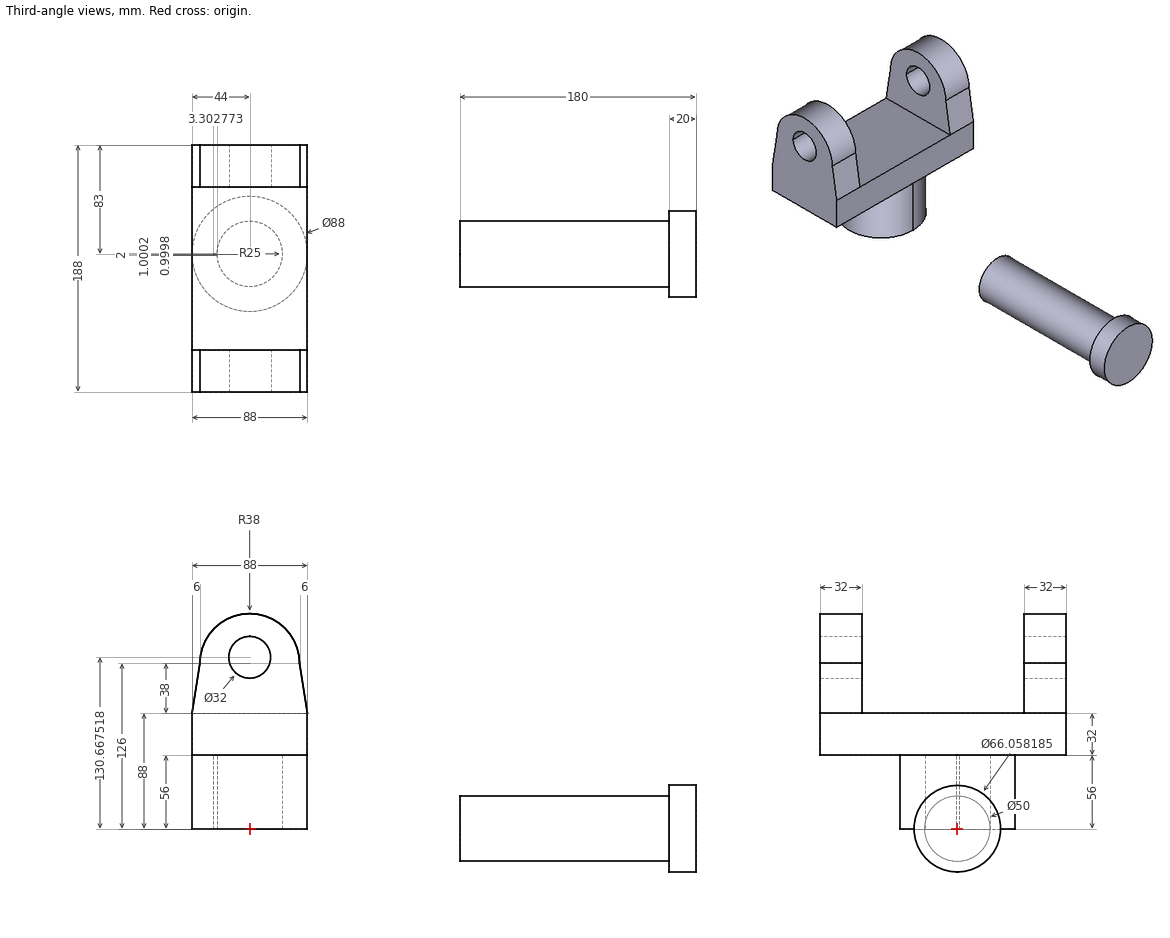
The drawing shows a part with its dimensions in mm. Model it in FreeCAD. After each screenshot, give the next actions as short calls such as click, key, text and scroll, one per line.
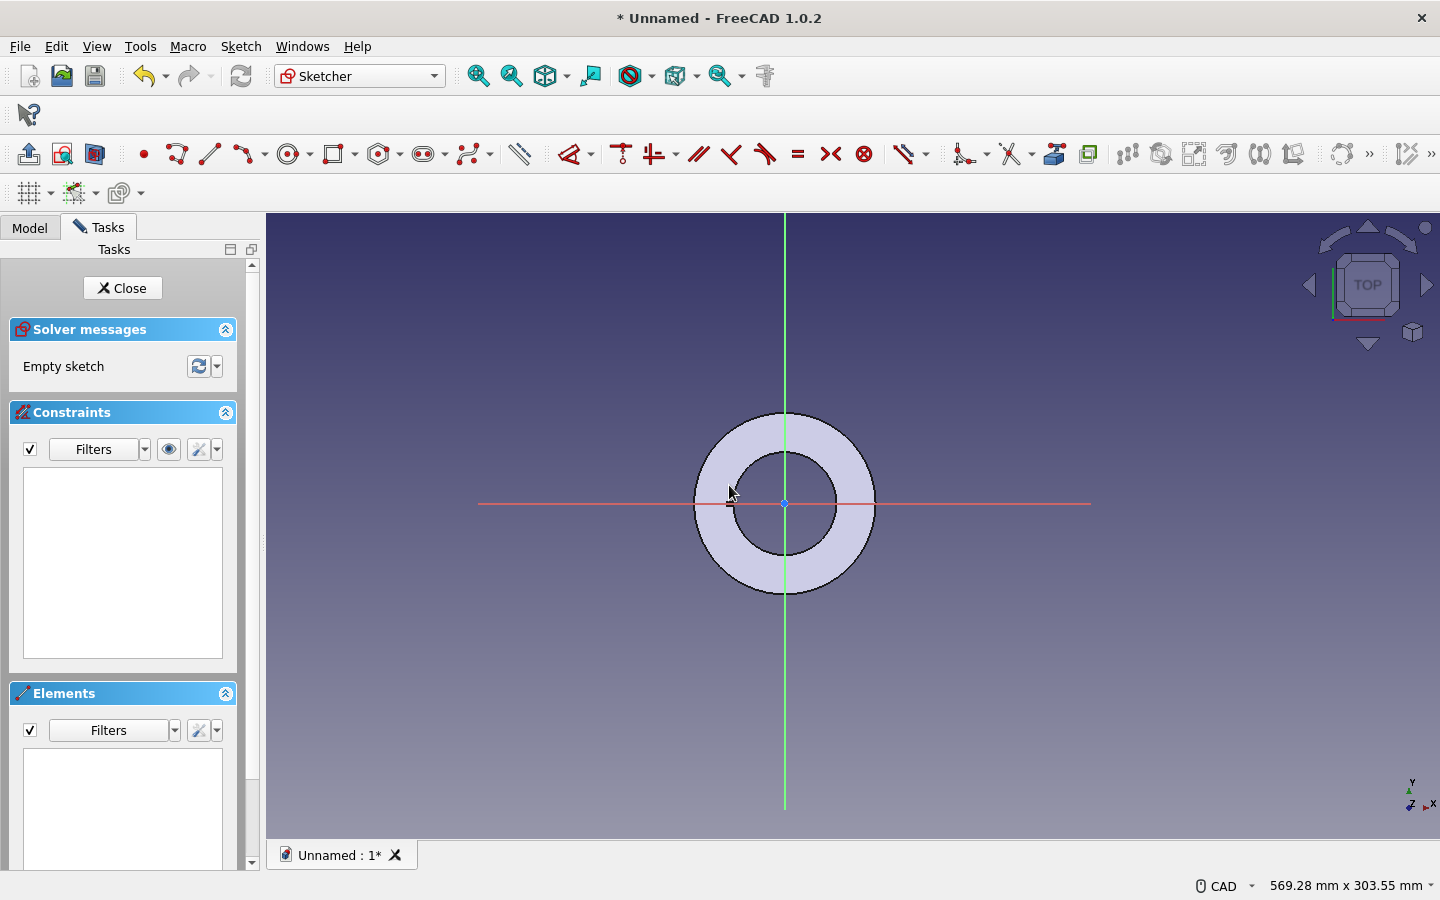
click(332, 154)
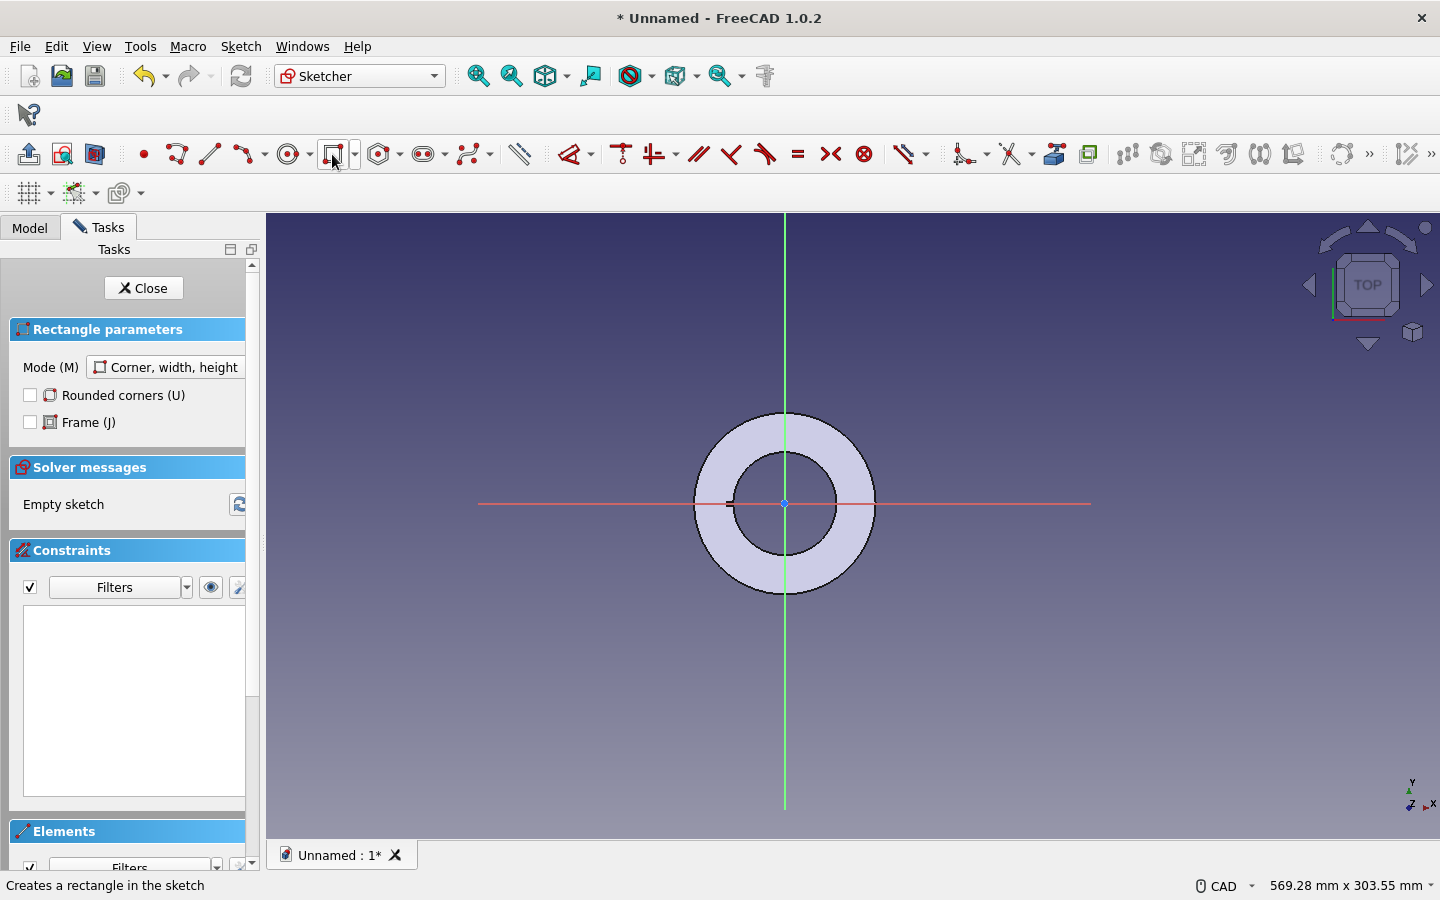
click(694, 332)
click(876, 720)
key(Escape)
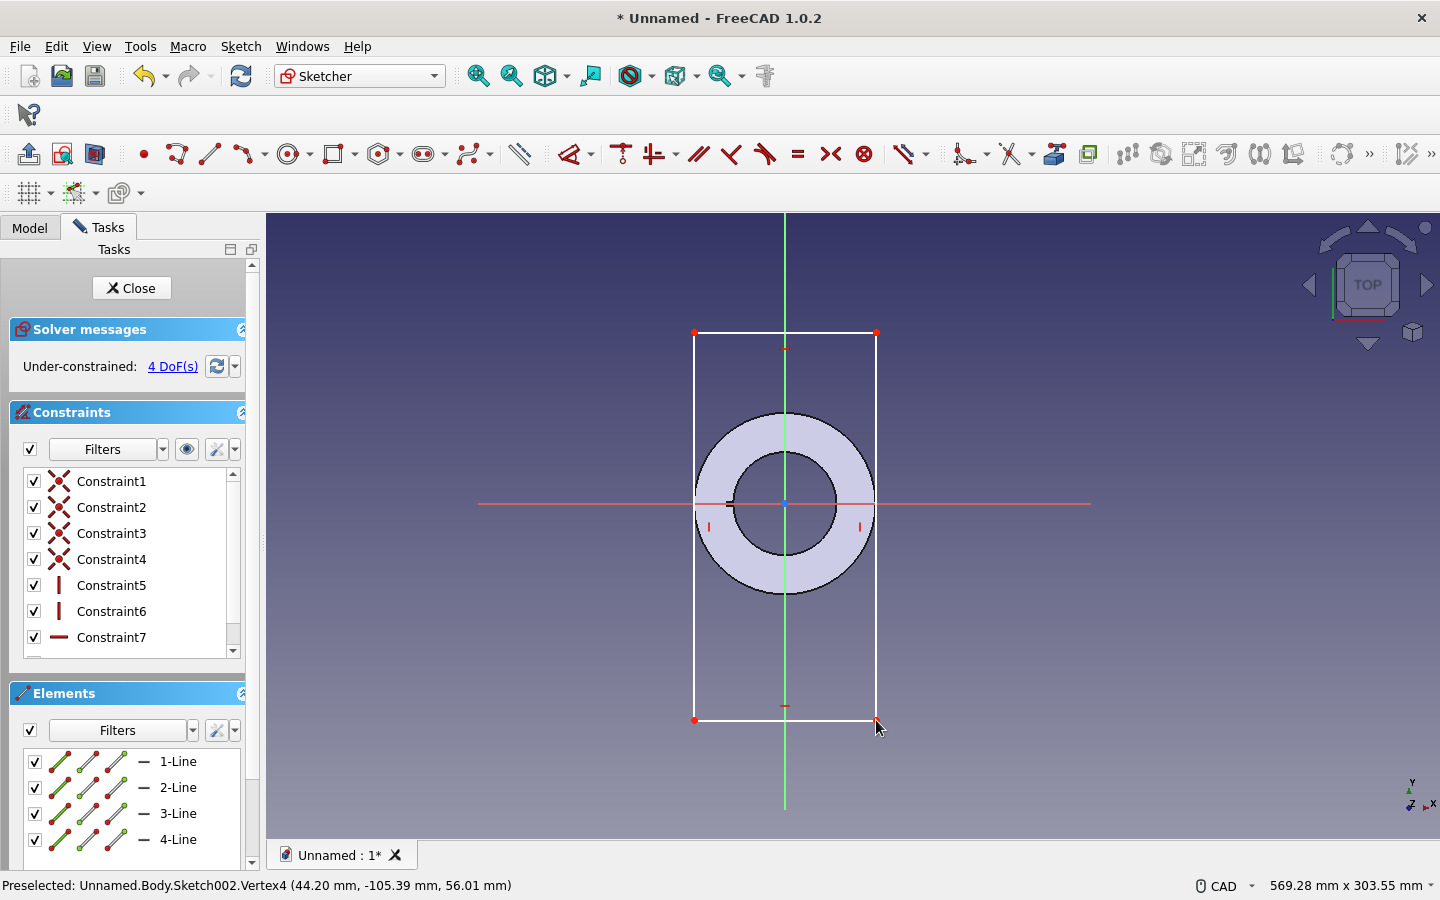
key(d)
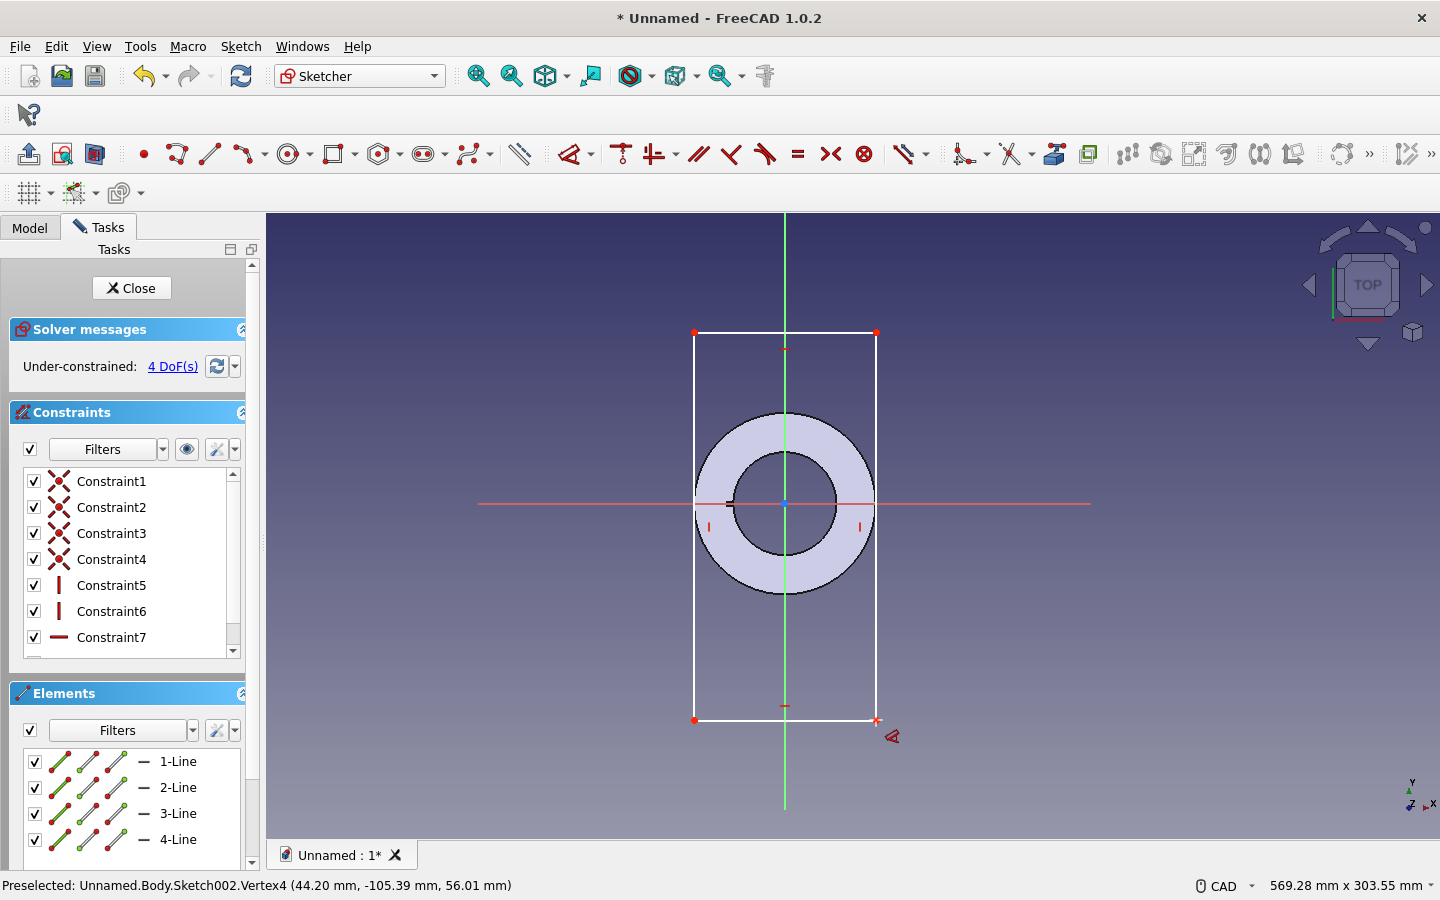
click(749, 721)
click(743, 755)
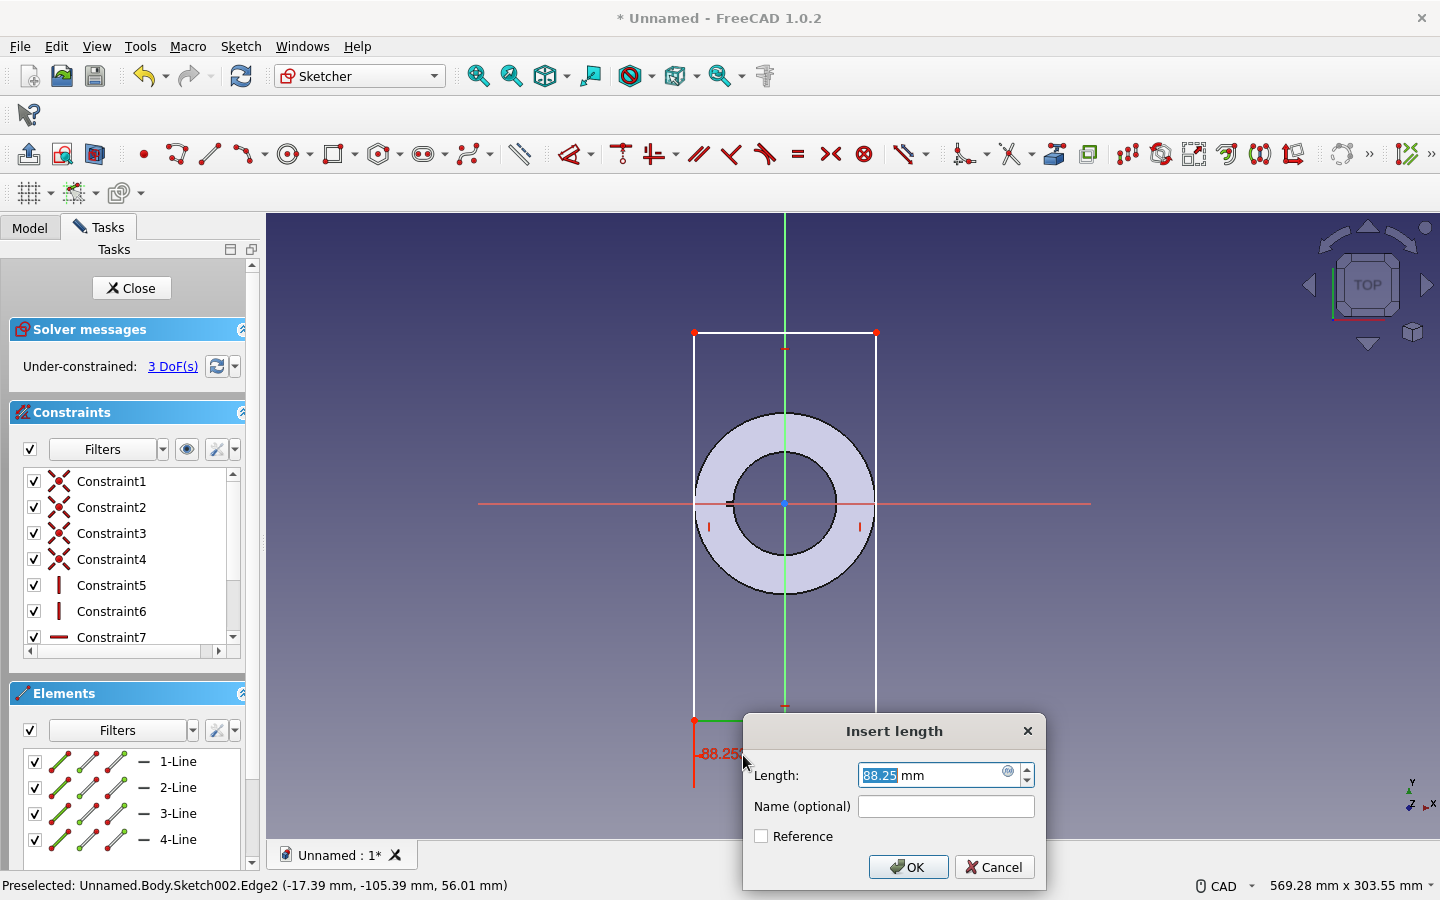
text(88)
key(Return)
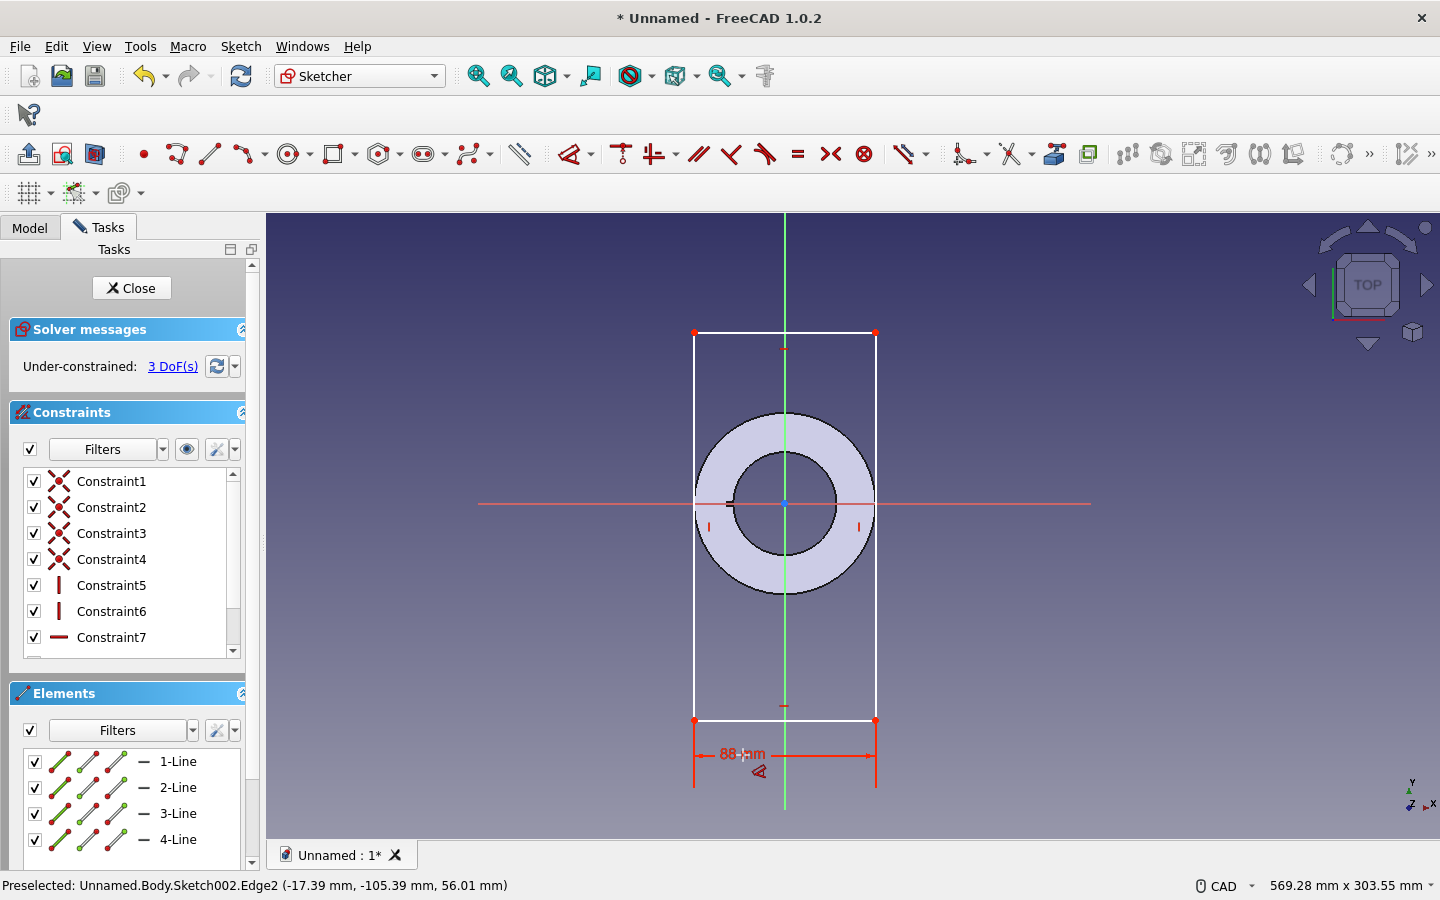
click(694, 449)
click(660, 527)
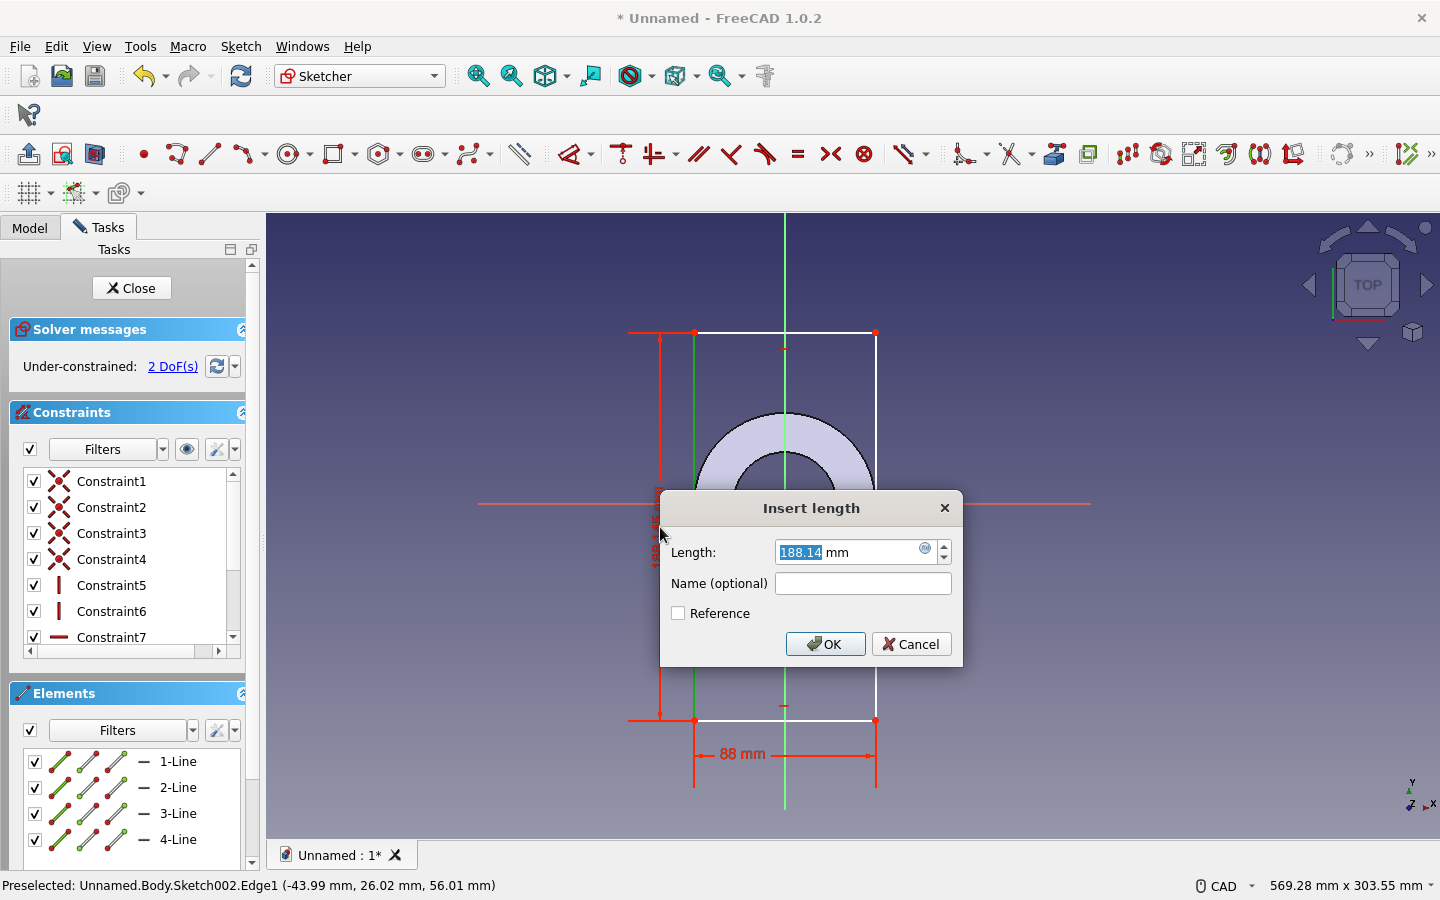
text(188)
key(Return)